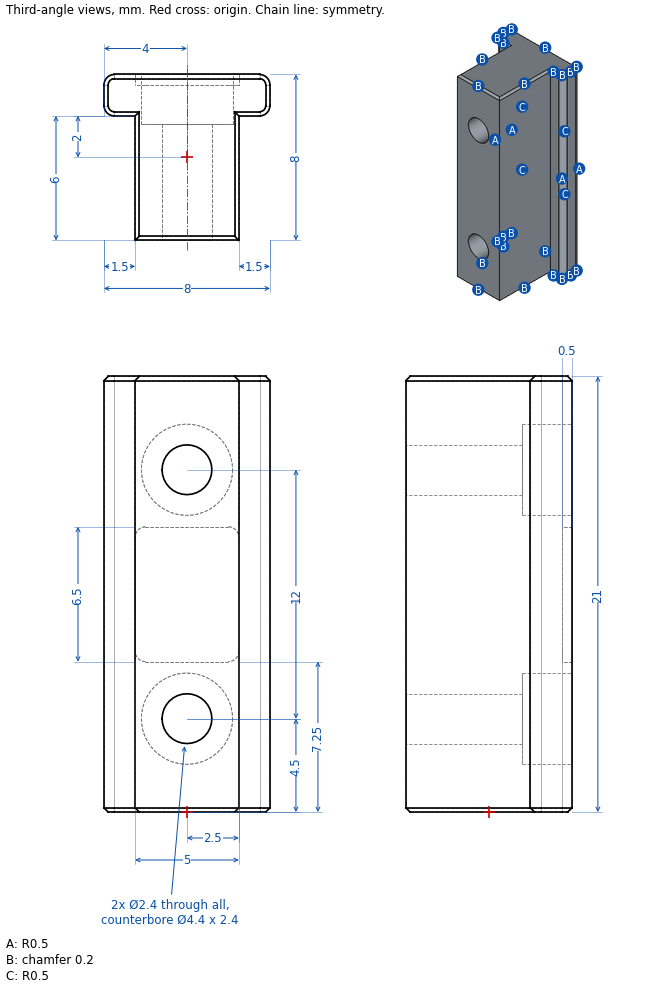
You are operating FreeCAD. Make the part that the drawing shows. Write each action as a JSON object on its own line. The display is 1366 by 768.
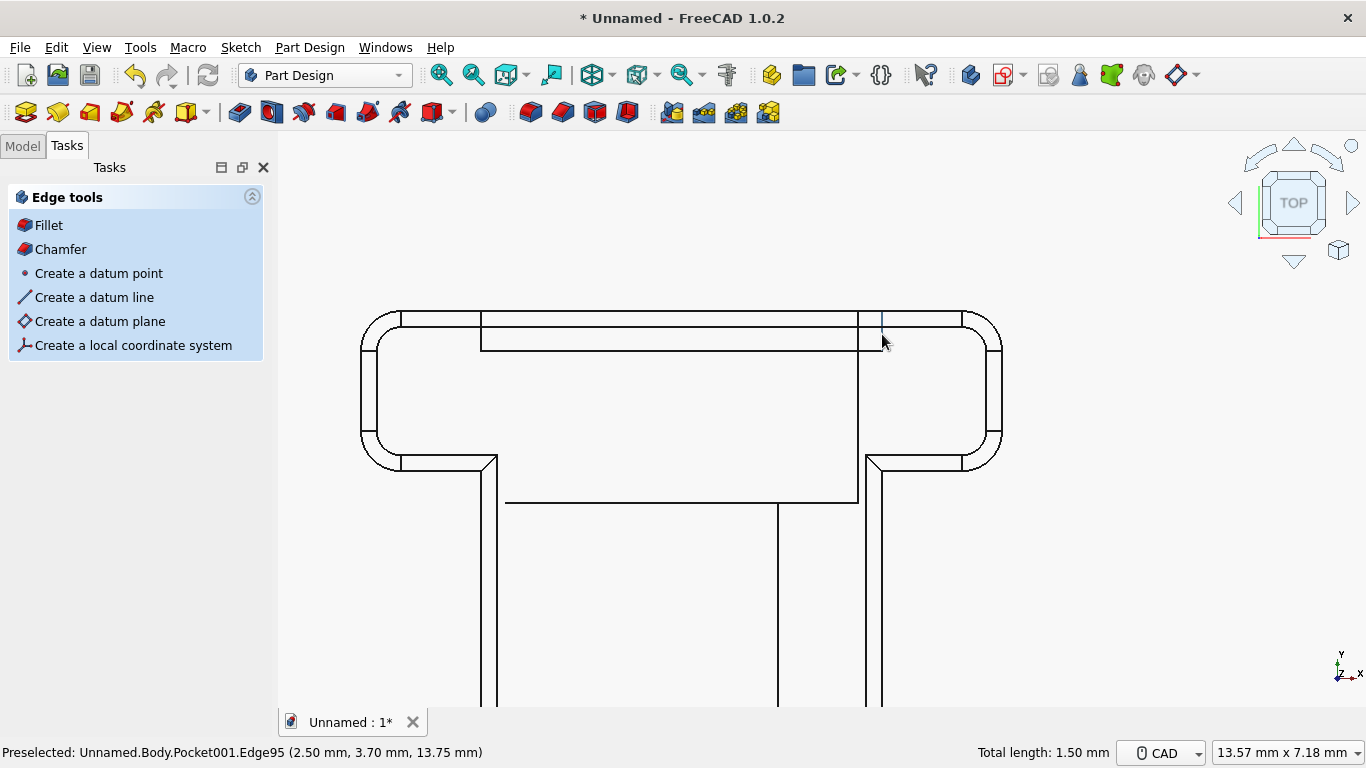
{"action": "left_click", "coordinate": [481, 334], "text": "ctrl"}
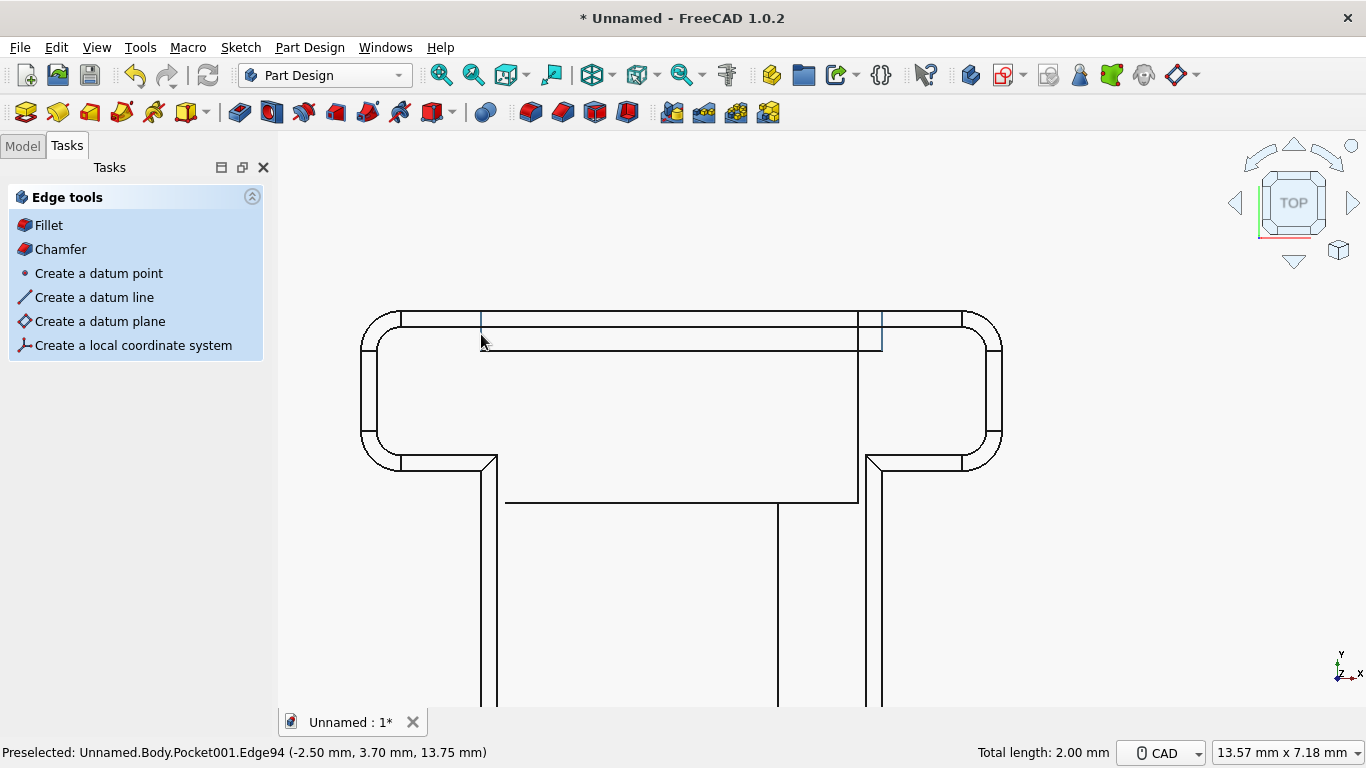
{"action": "key", "text": "v 1"}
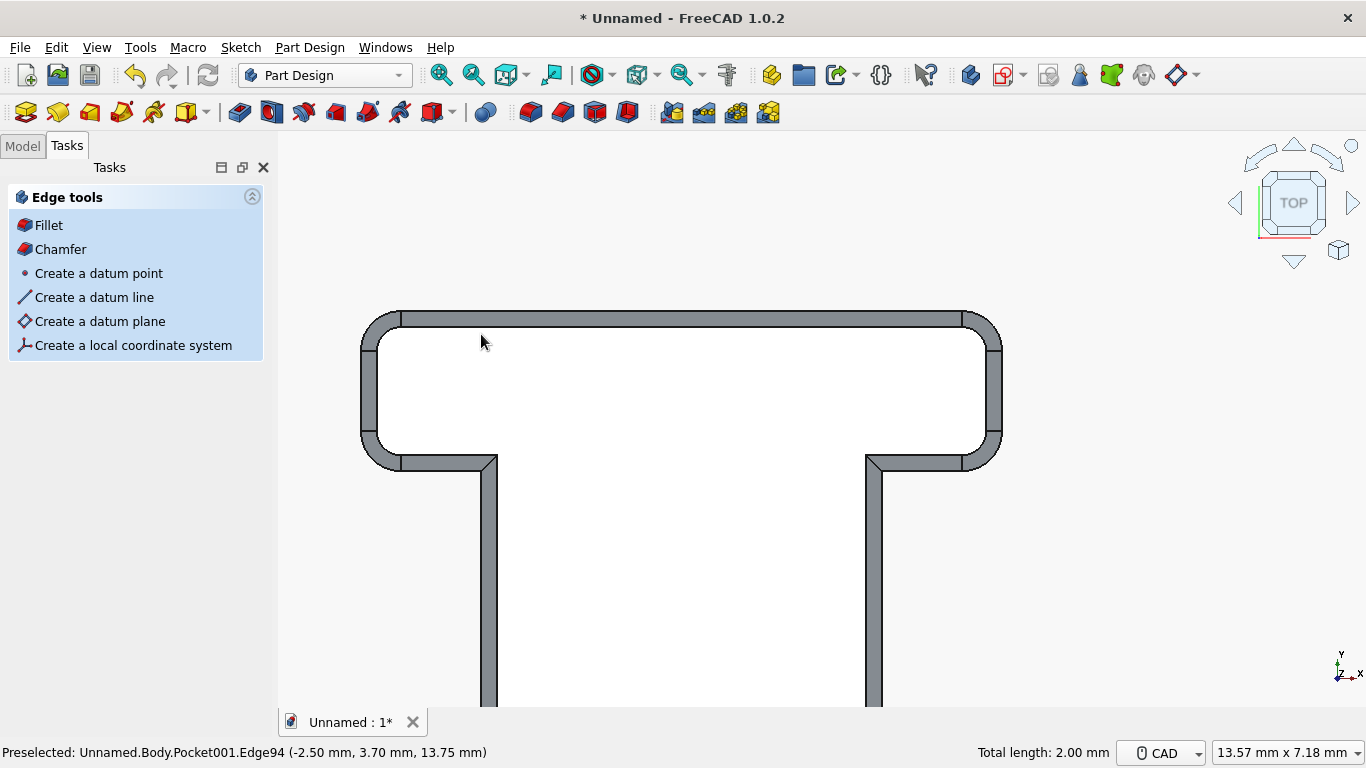
{"action": "left_click", "coordinate": [532, 112]}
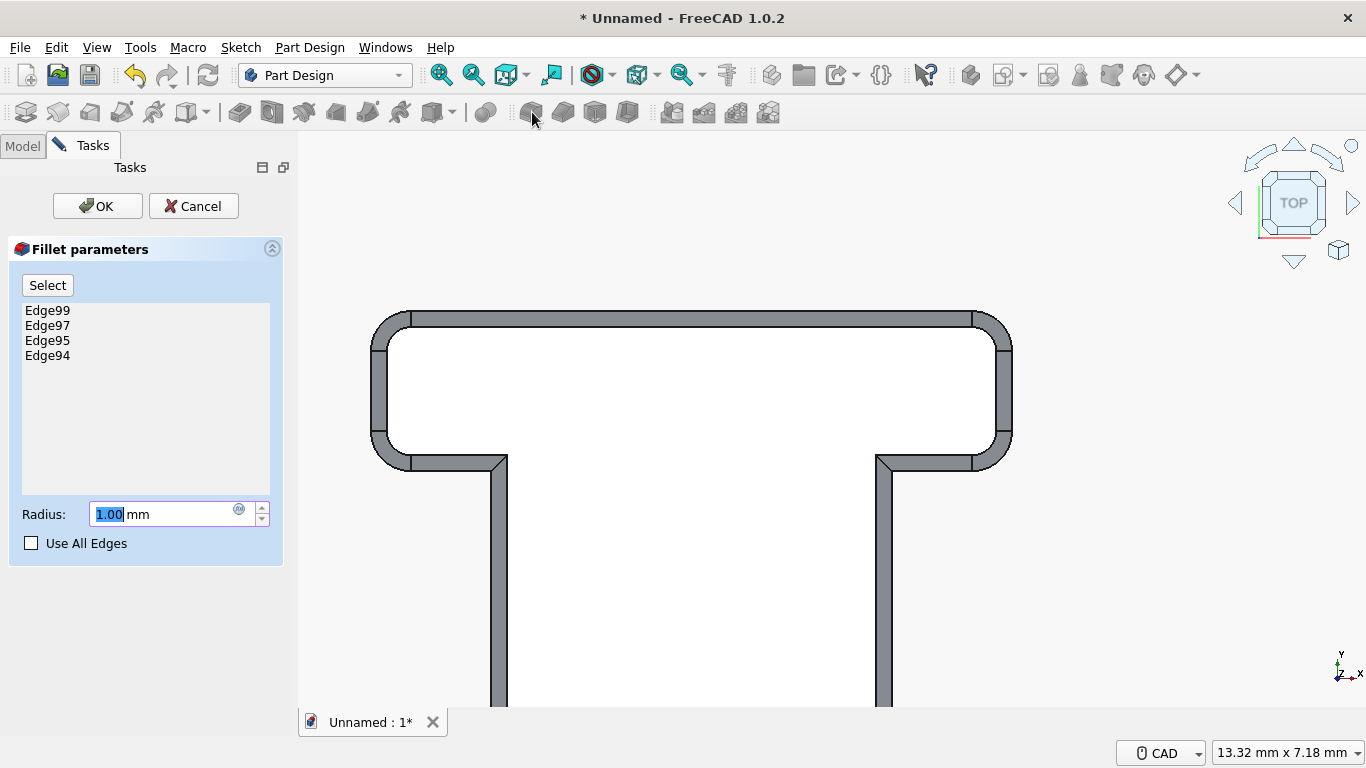
{"action": "type", "text": "0.5"}
{"action": "key", "text": "Tab"}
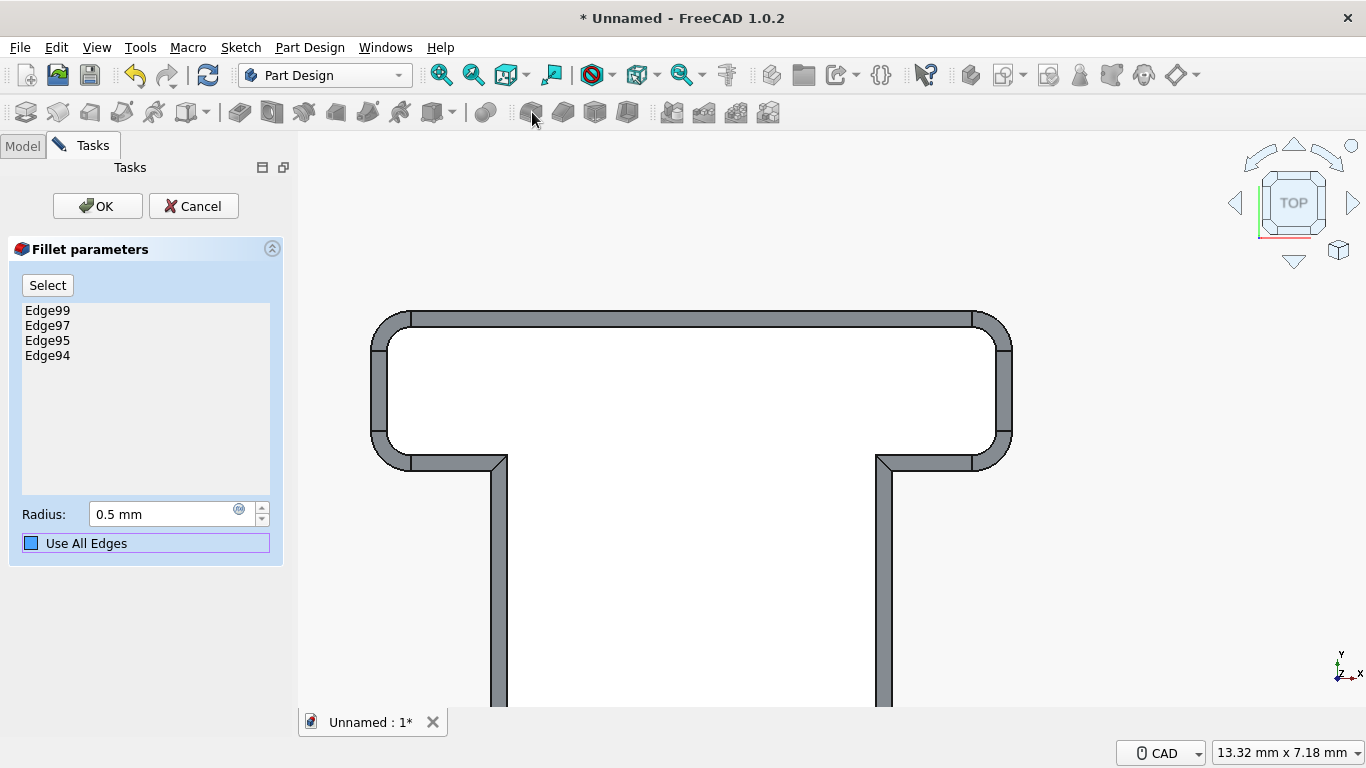
{"action": "left_click", "coordinate": [98, 206]}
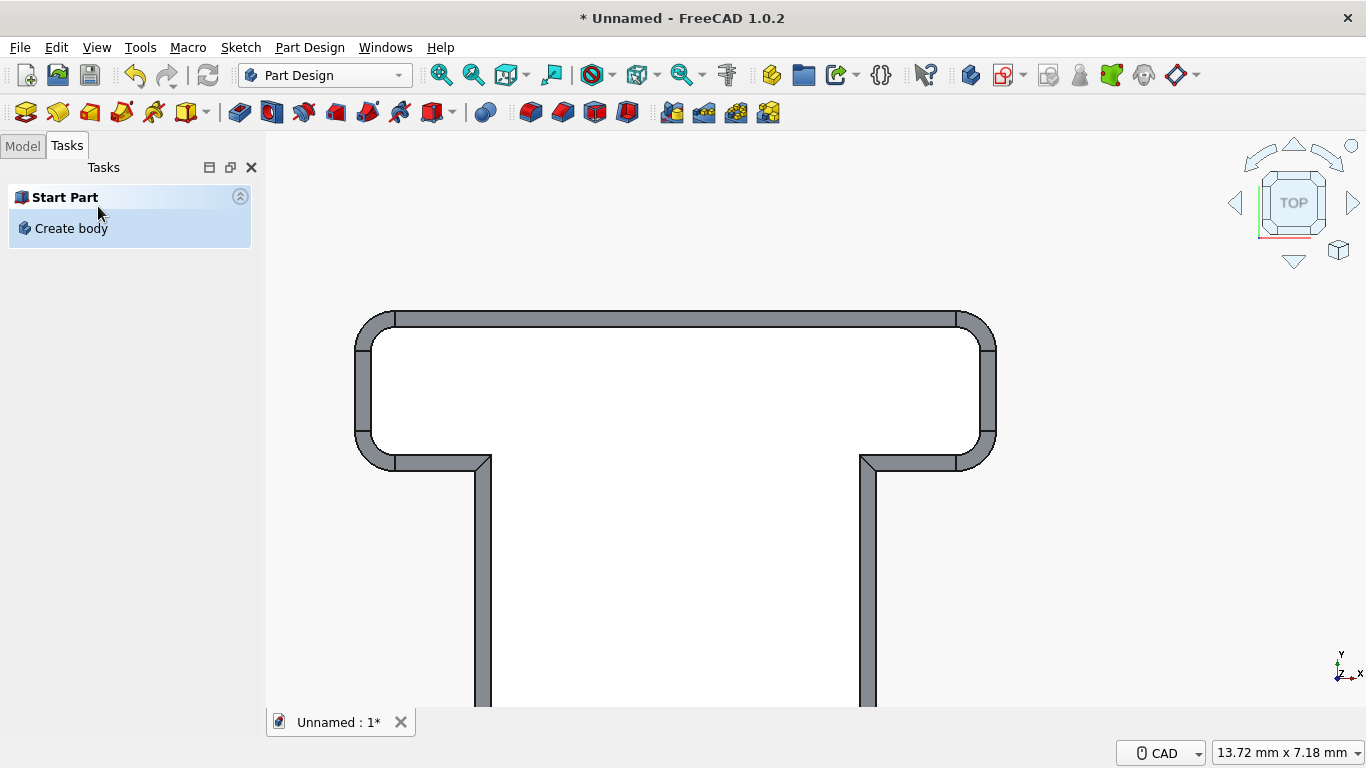
{"action": "key", "text": "0"}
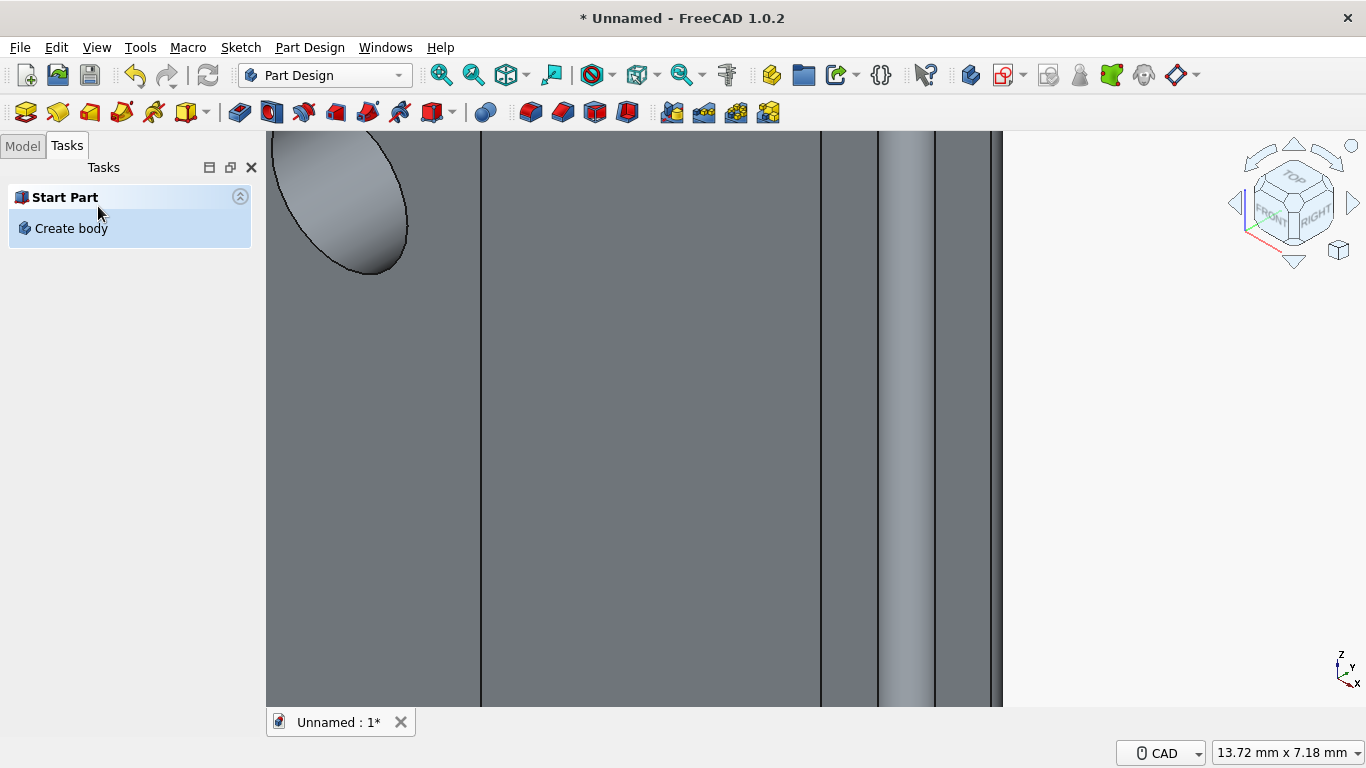
{"action": "left_click", "coordinate": [442, 76]}